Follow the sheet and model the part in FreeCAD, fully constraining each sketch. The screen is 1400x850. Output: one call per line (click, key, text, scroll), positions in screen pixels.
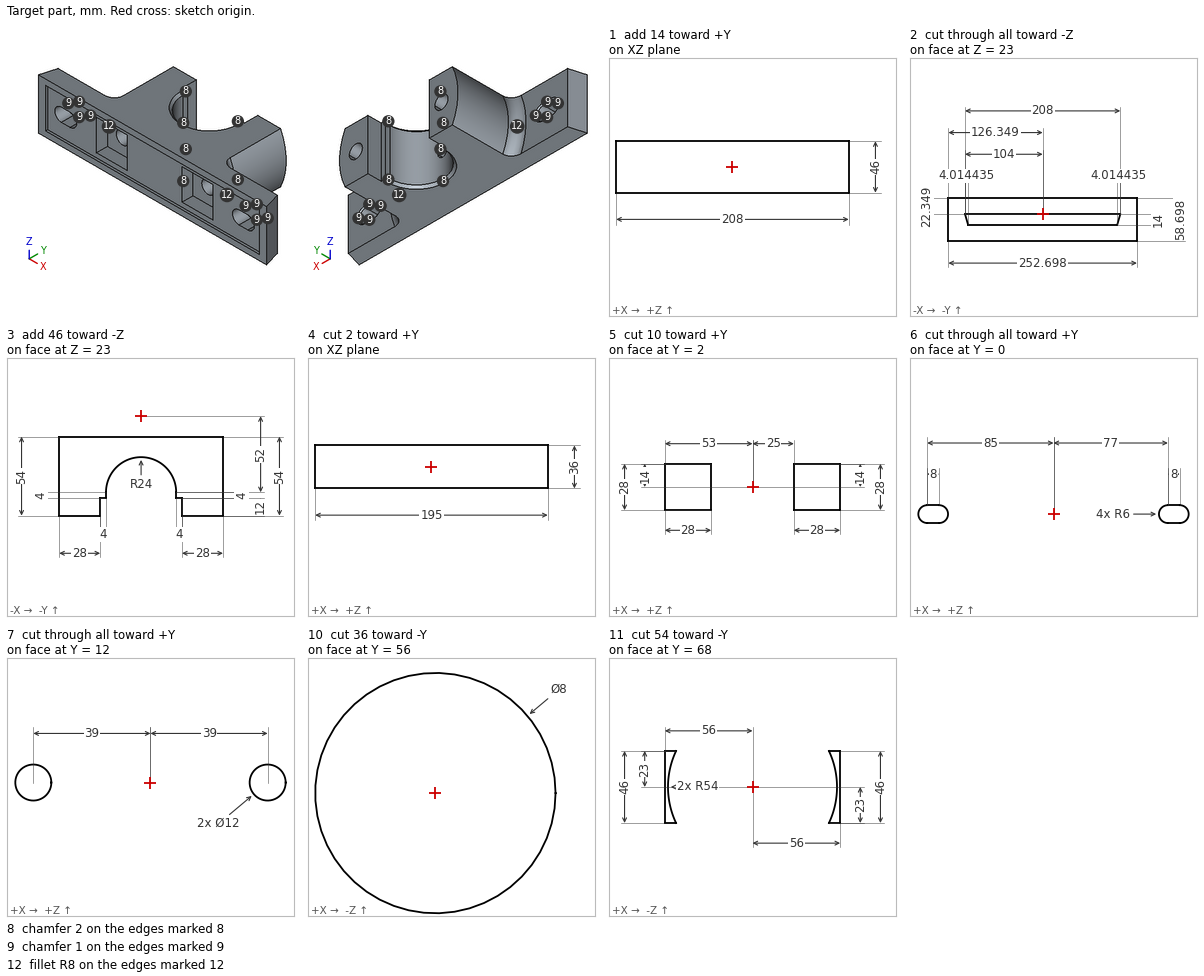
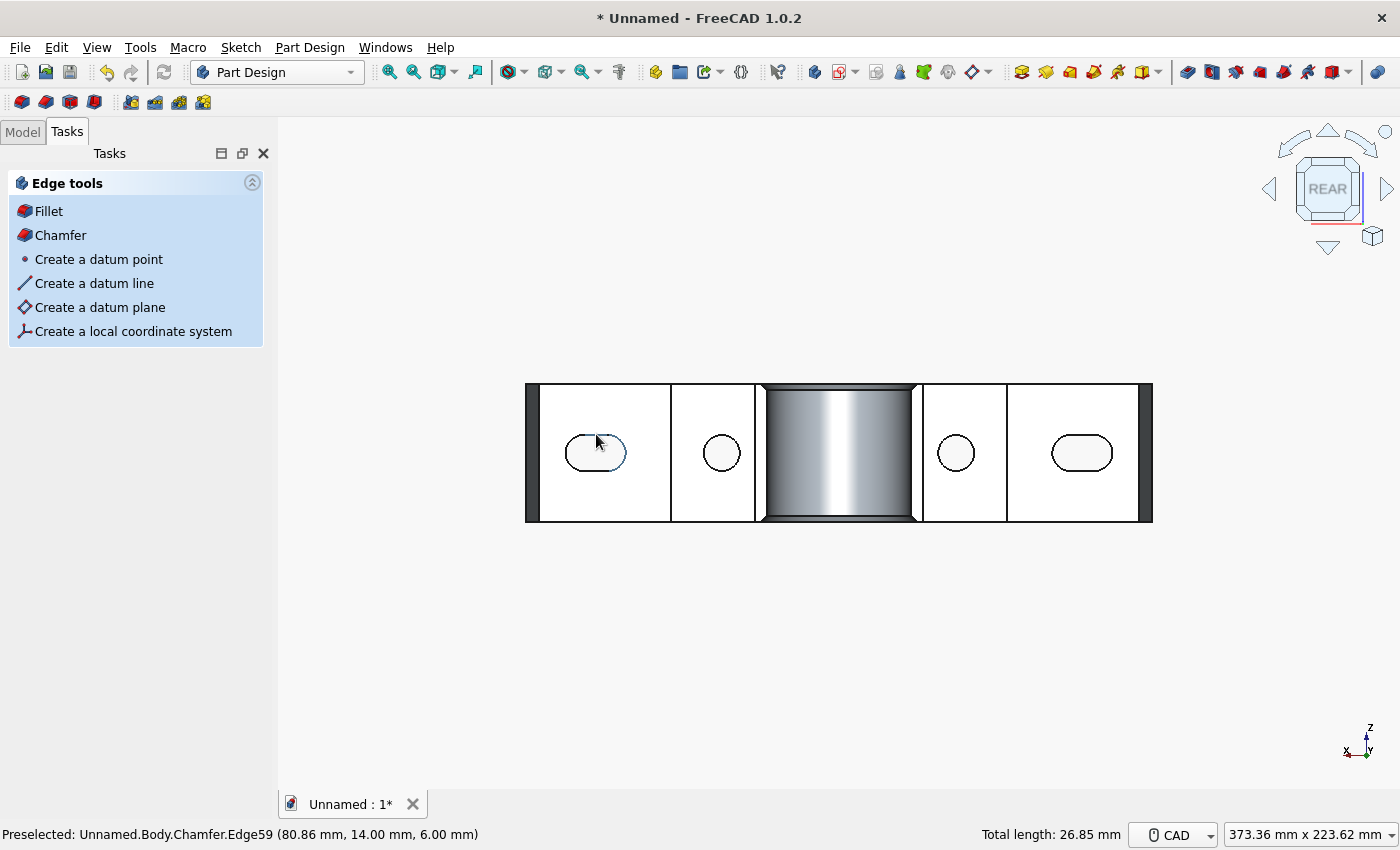
click(566, 452, ctrl)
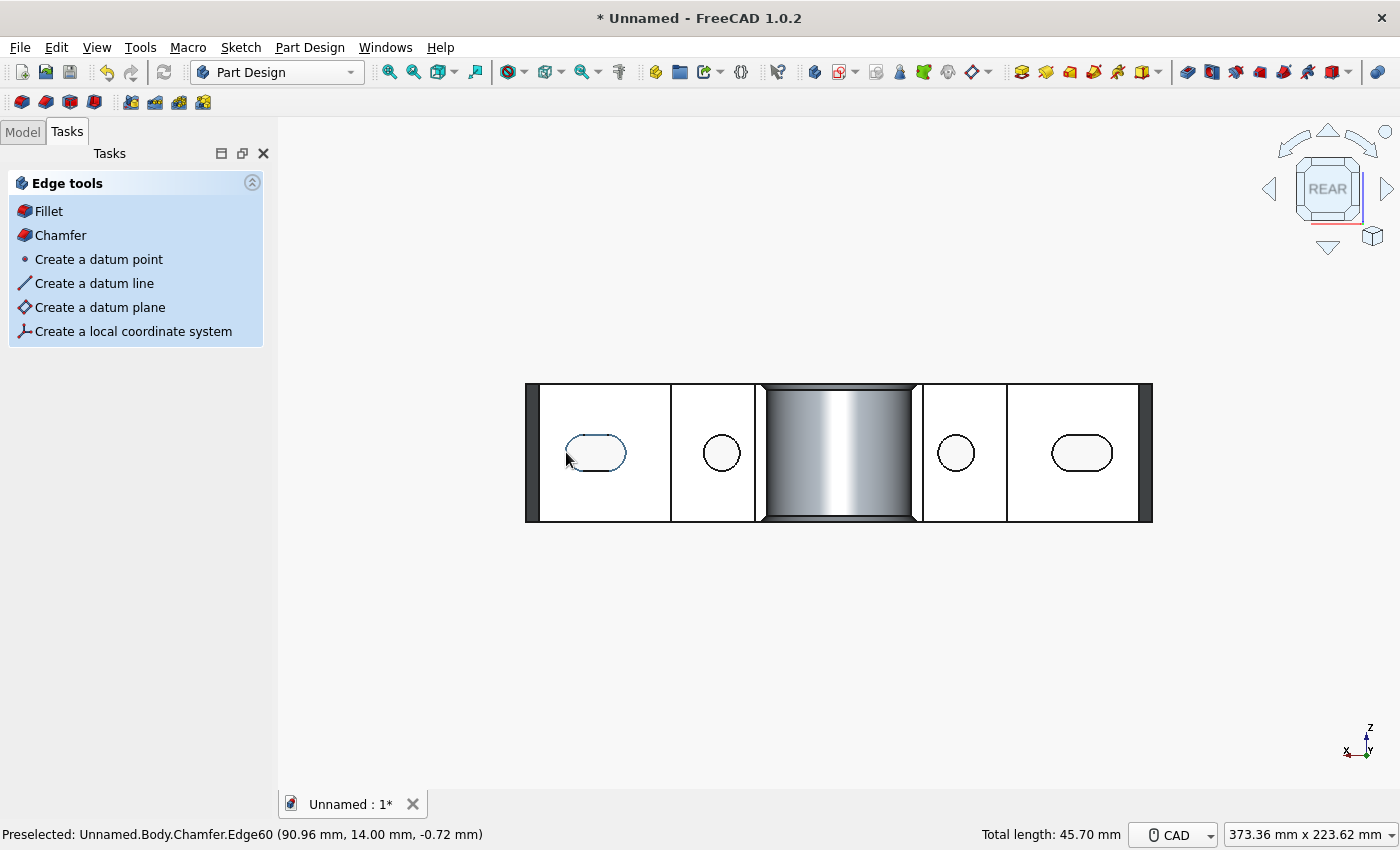
click(1052, 452, ctrl)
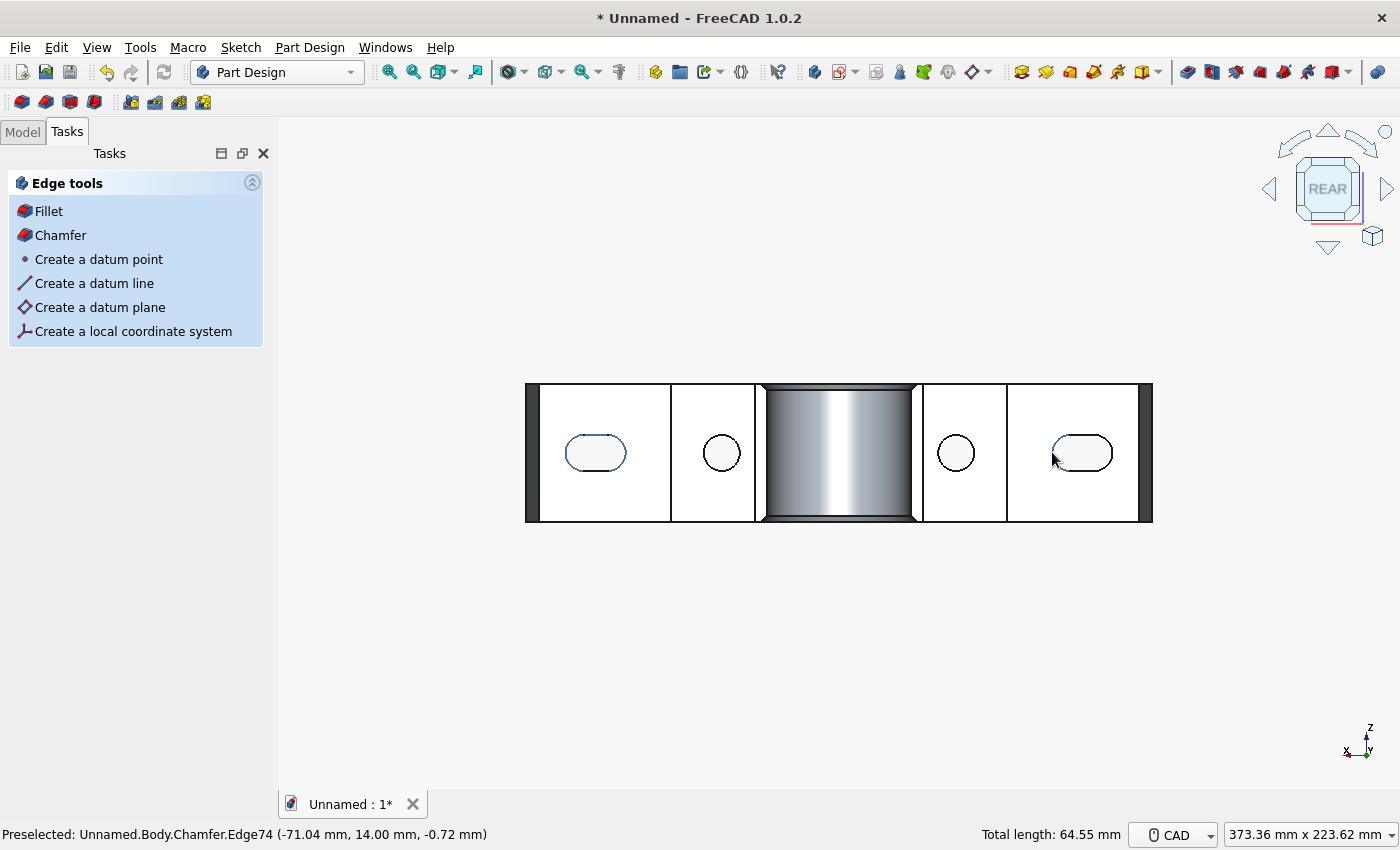
click(1112, 452, ctrl)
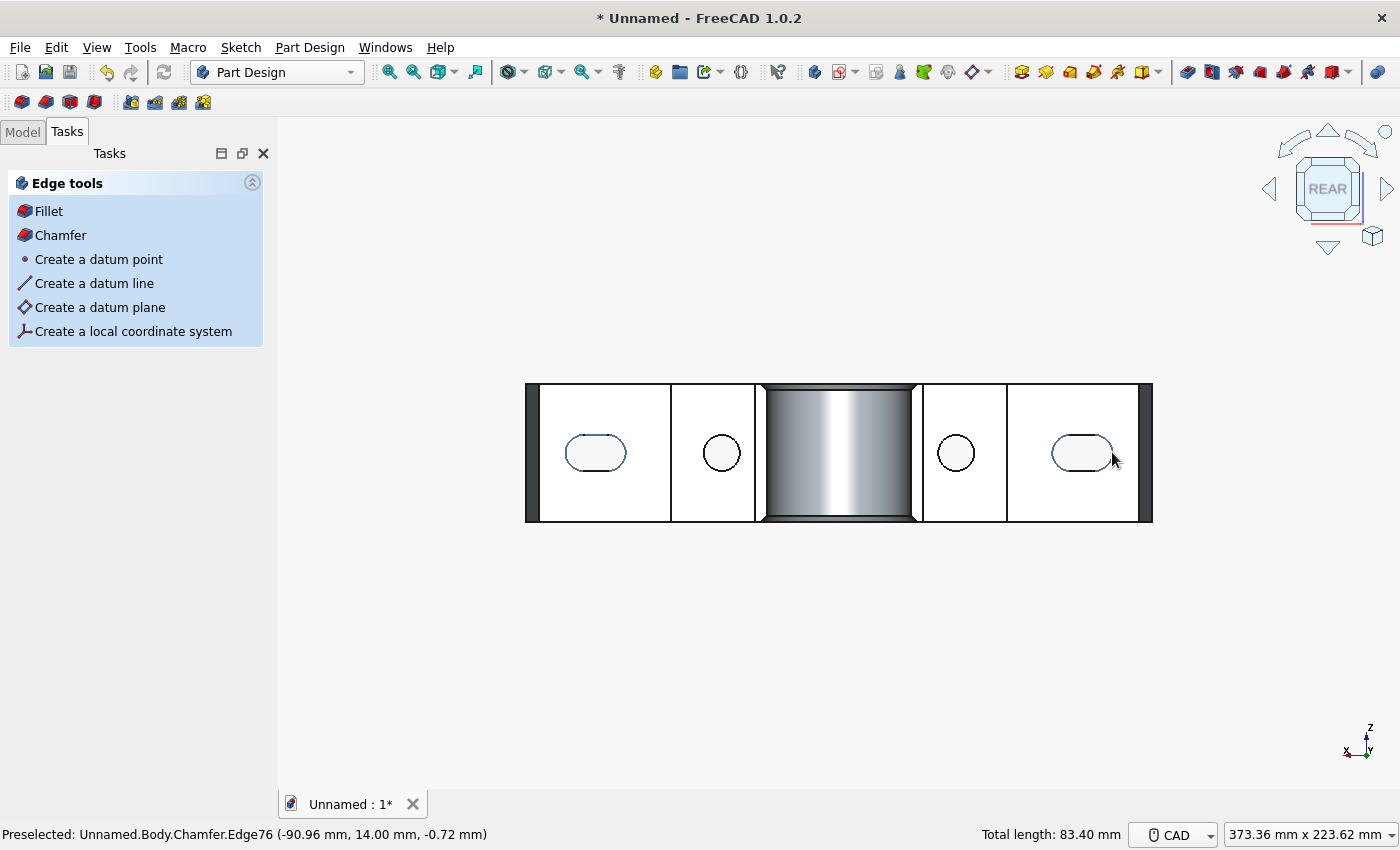
click(1082, 434, ctrl)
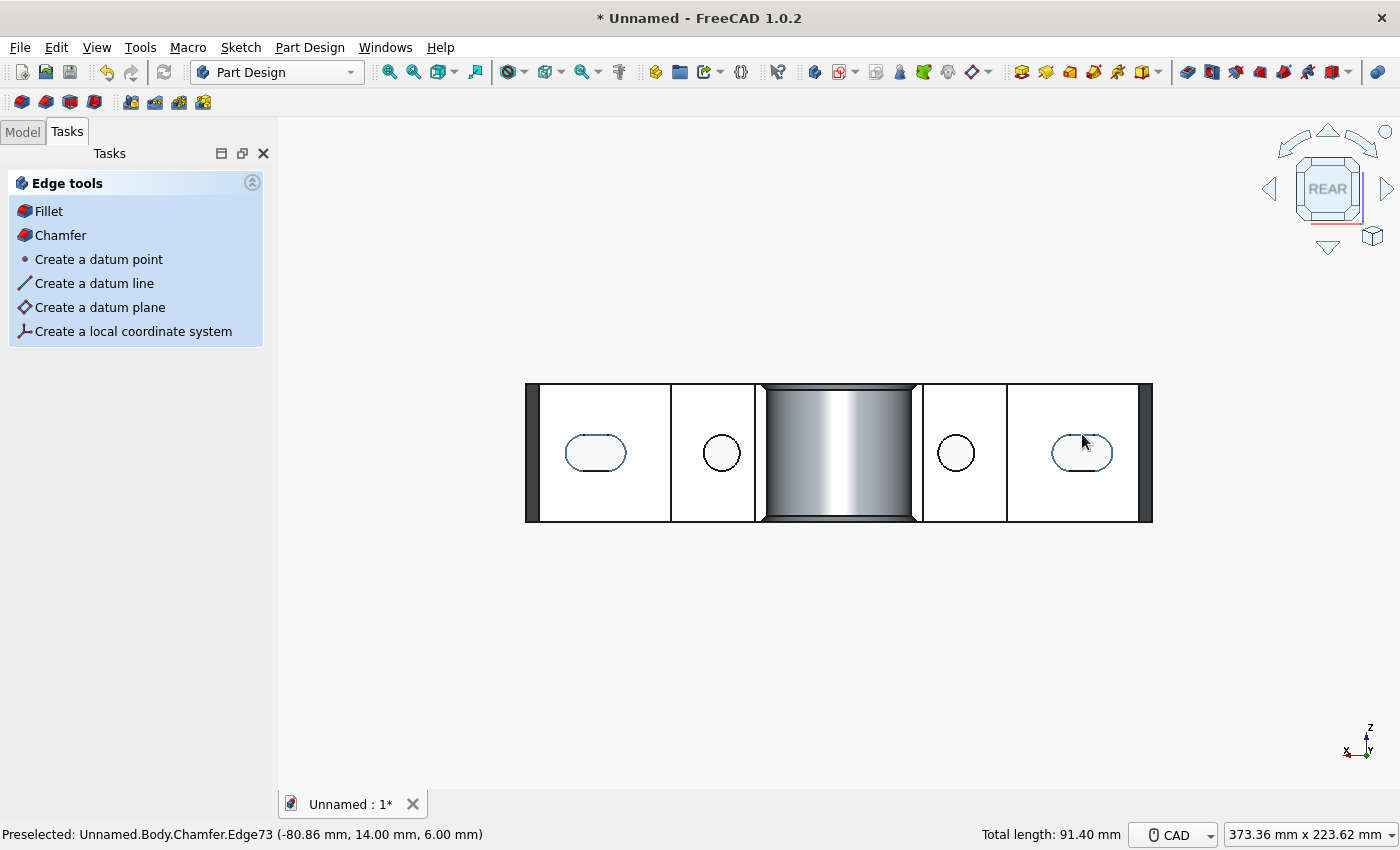
key(0)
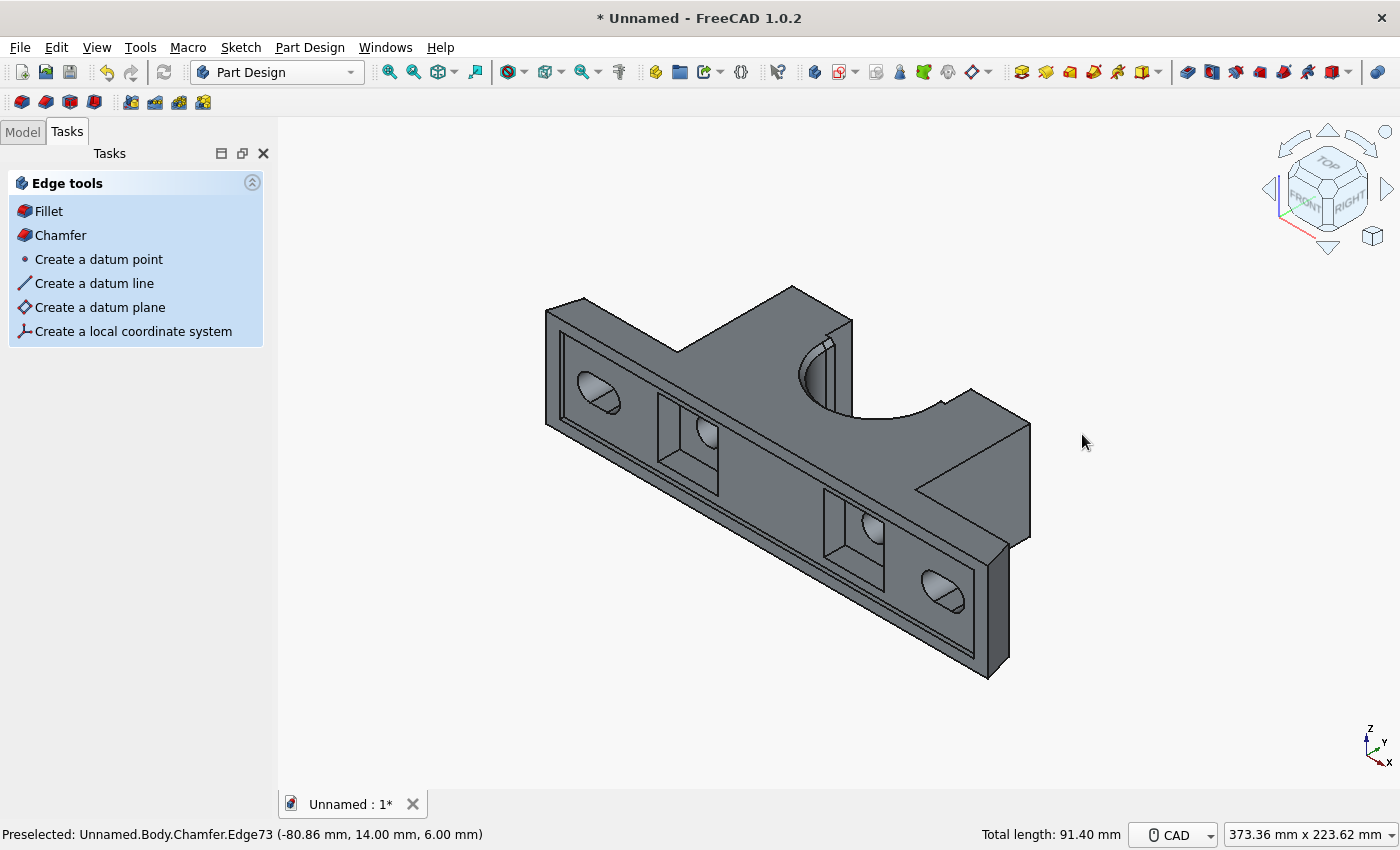
key(2)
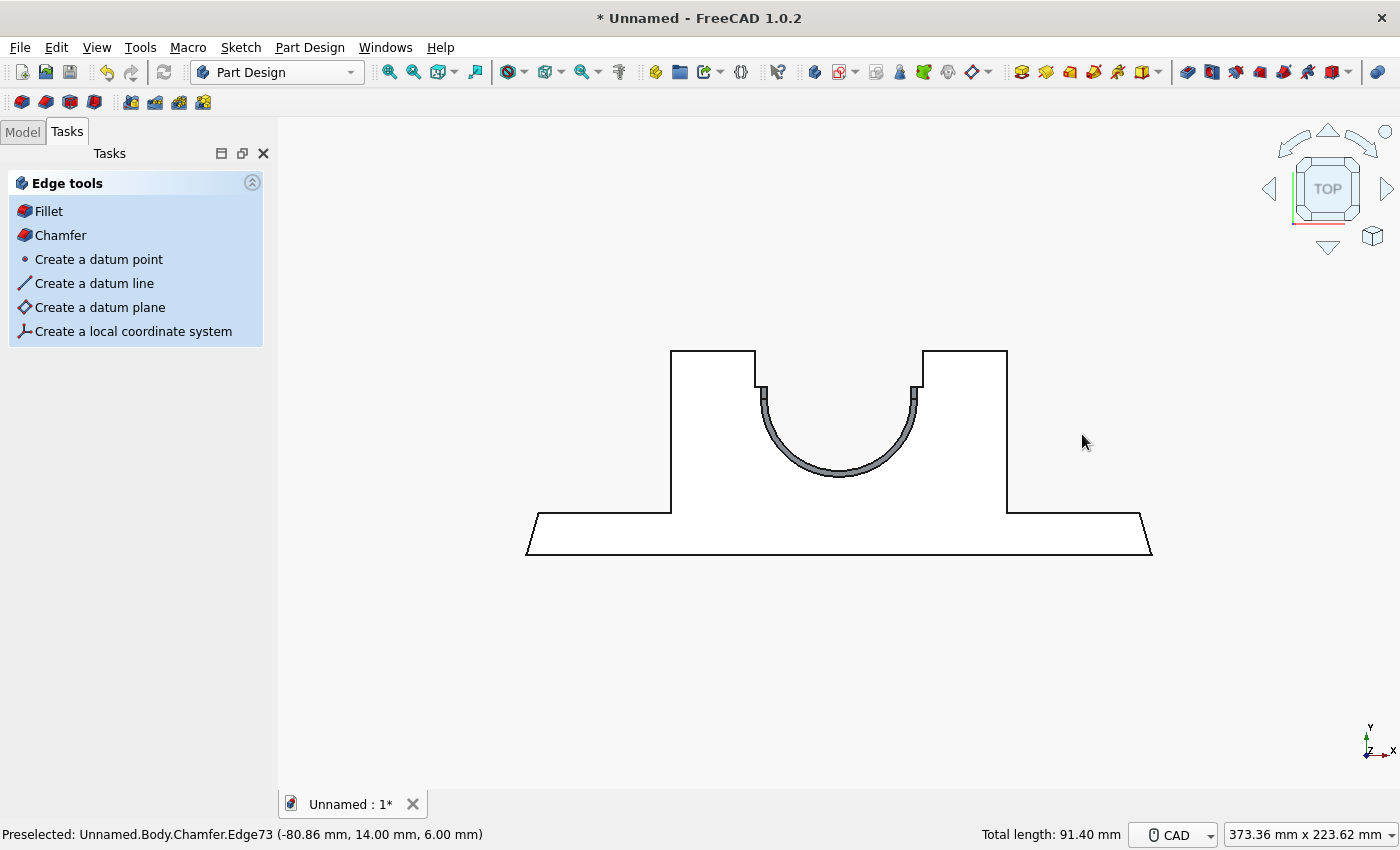
key(1)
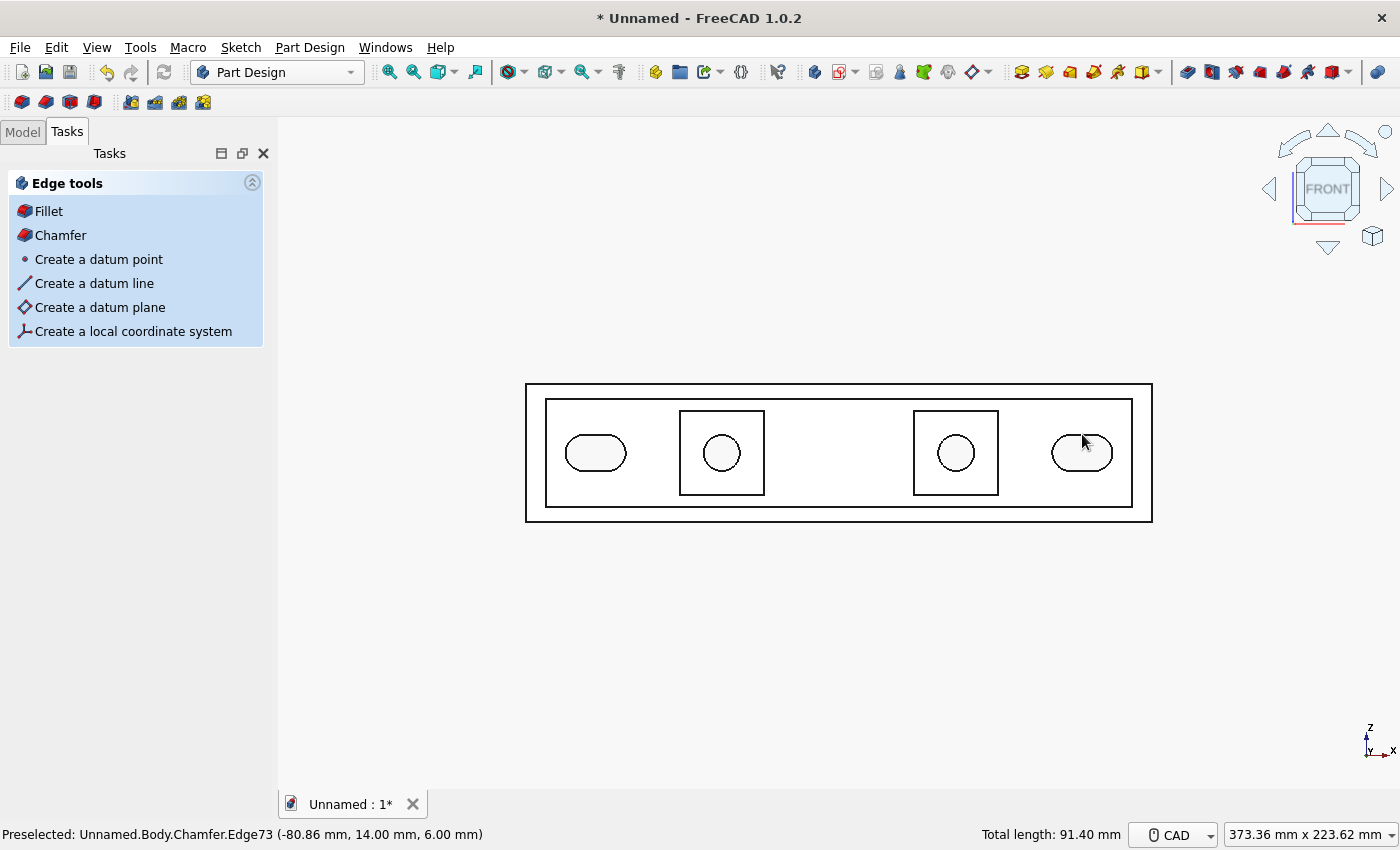
key(3)